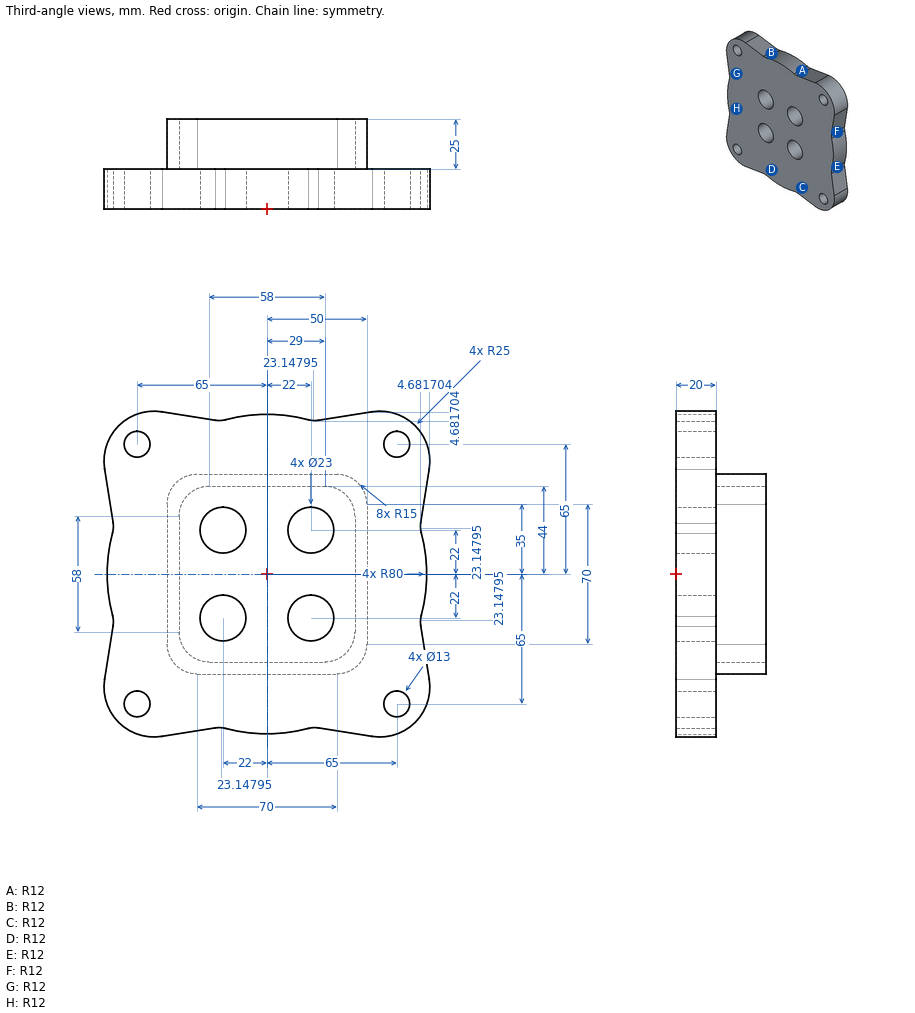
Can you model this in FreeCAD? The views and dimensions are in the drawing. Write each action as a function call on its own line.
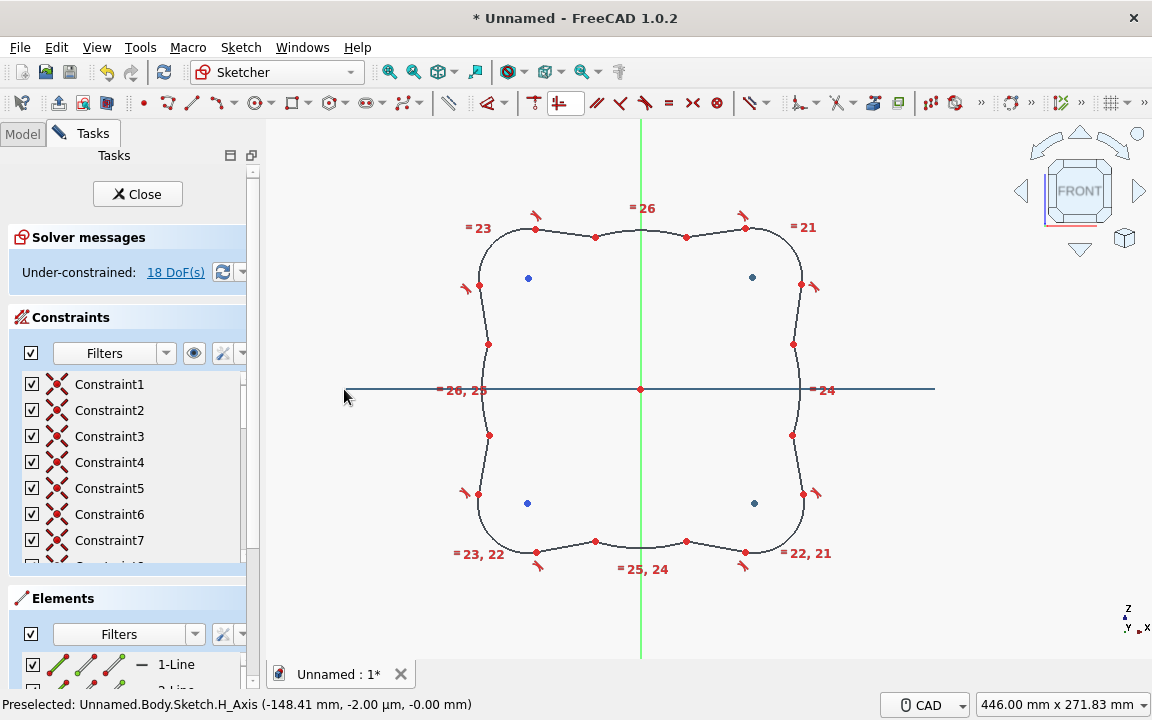
click(694, 104)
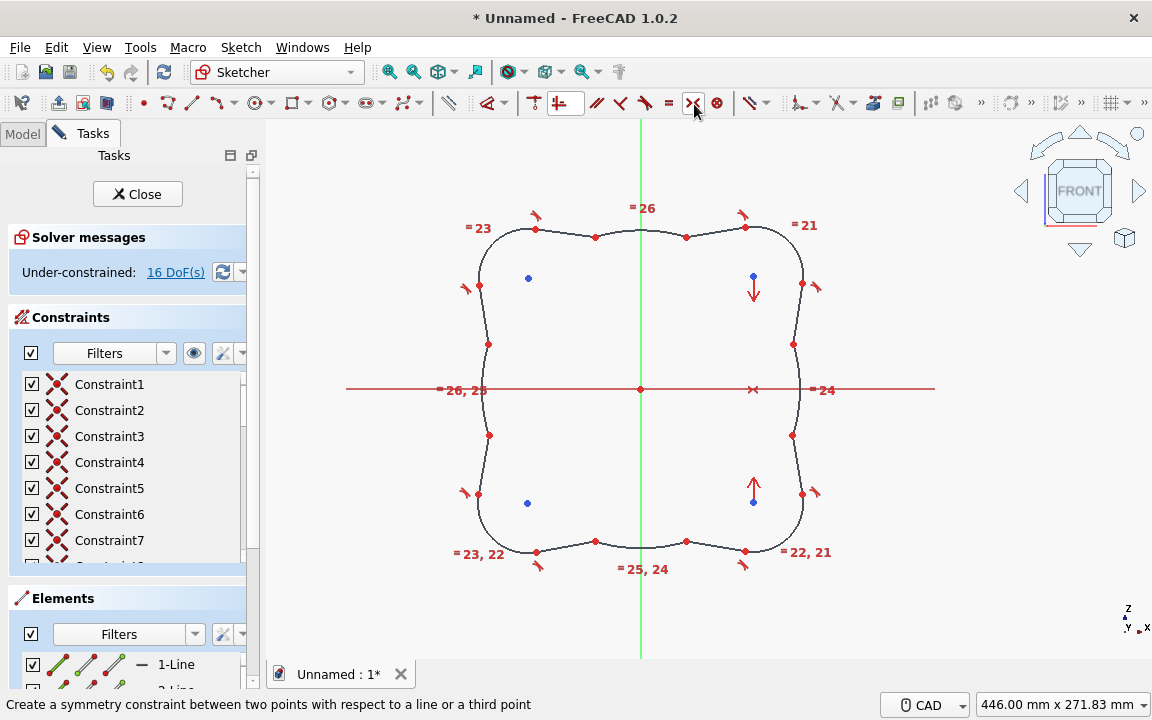
click(754, 502)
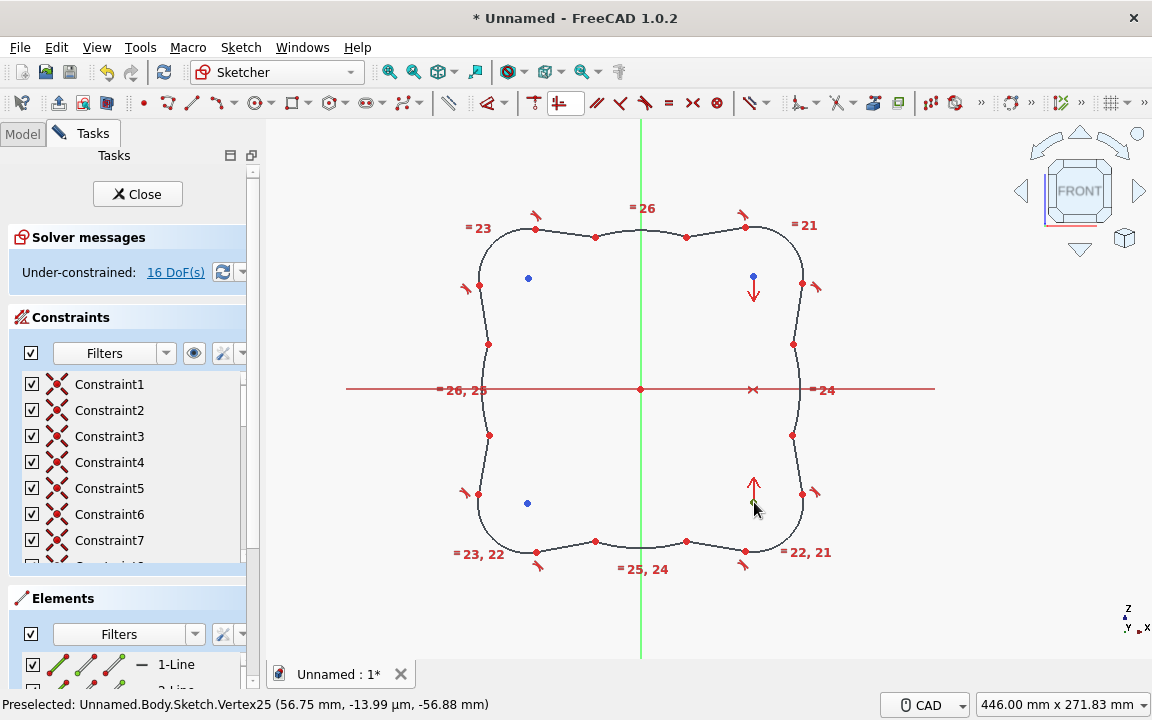
click(528, 504)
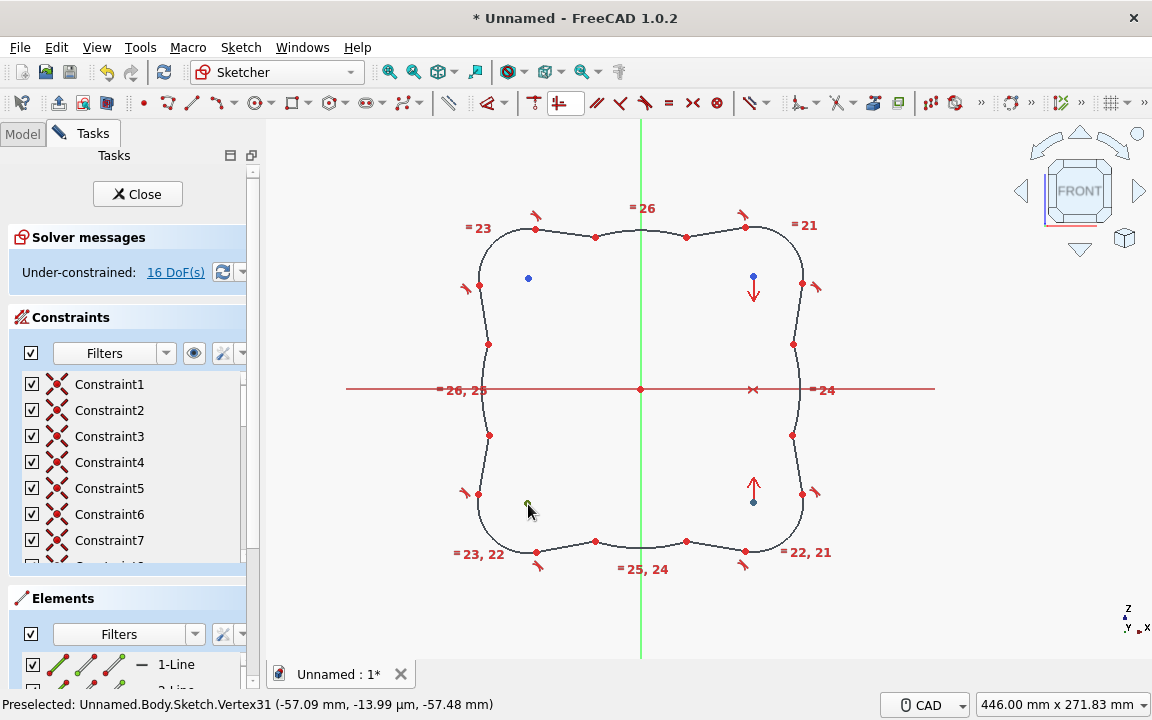
click(641, 596)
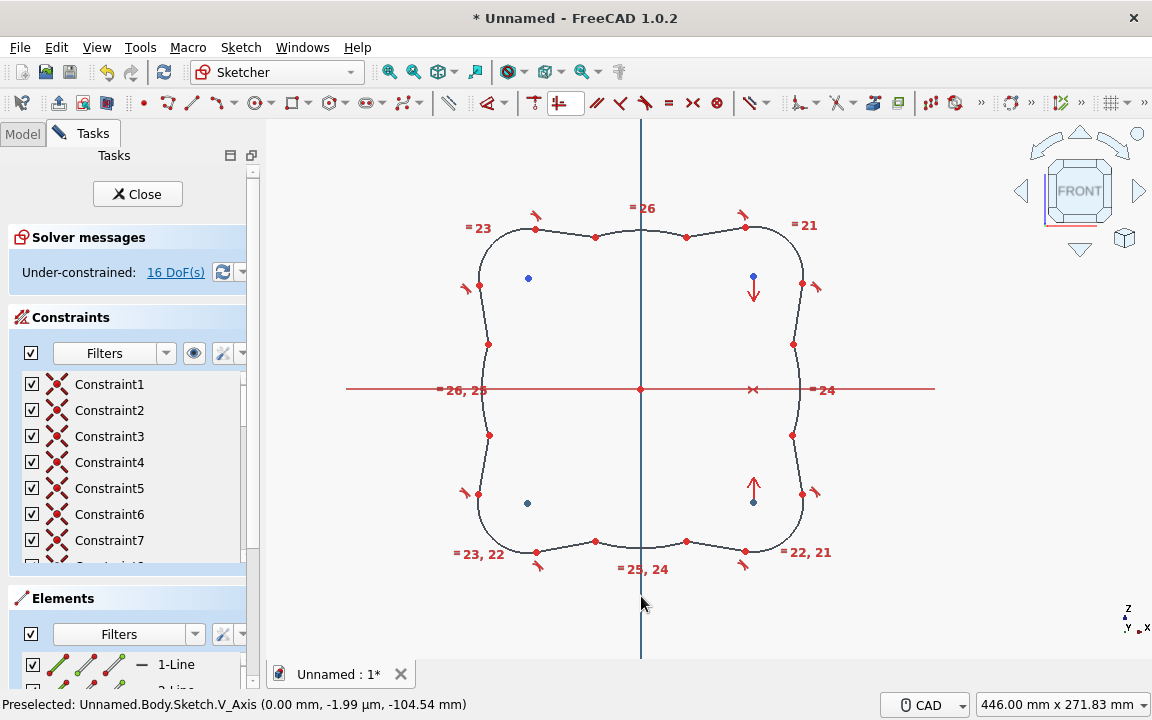
click(694, 104)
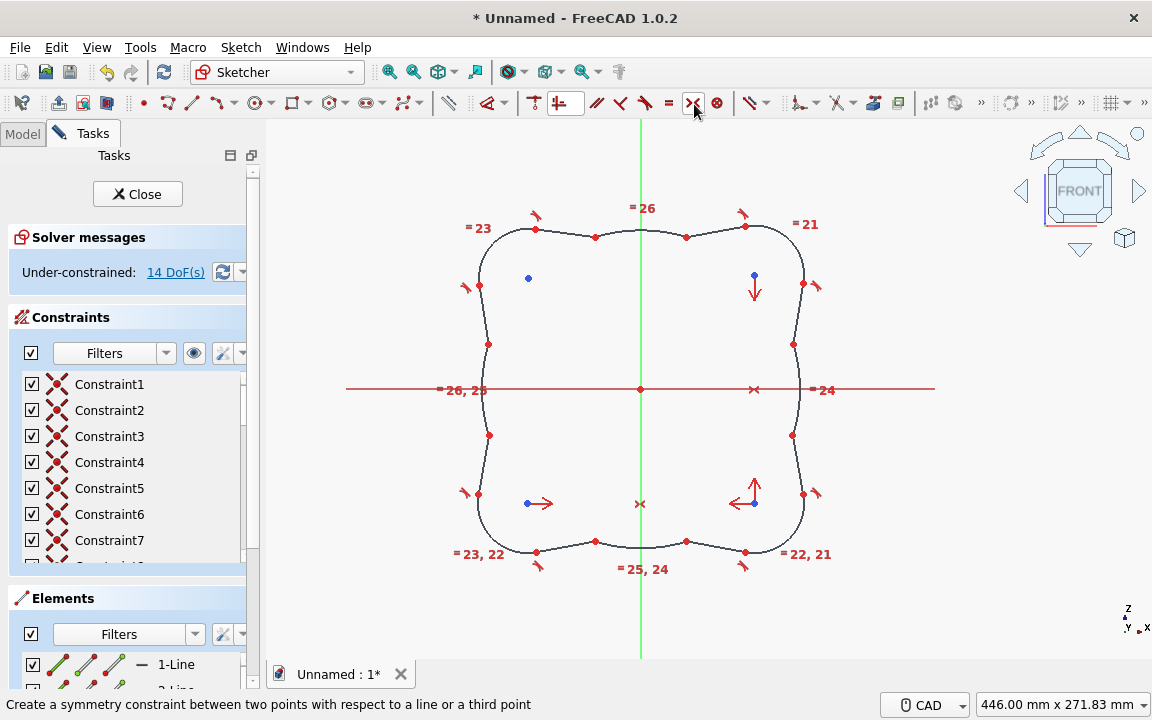
click(755, 275)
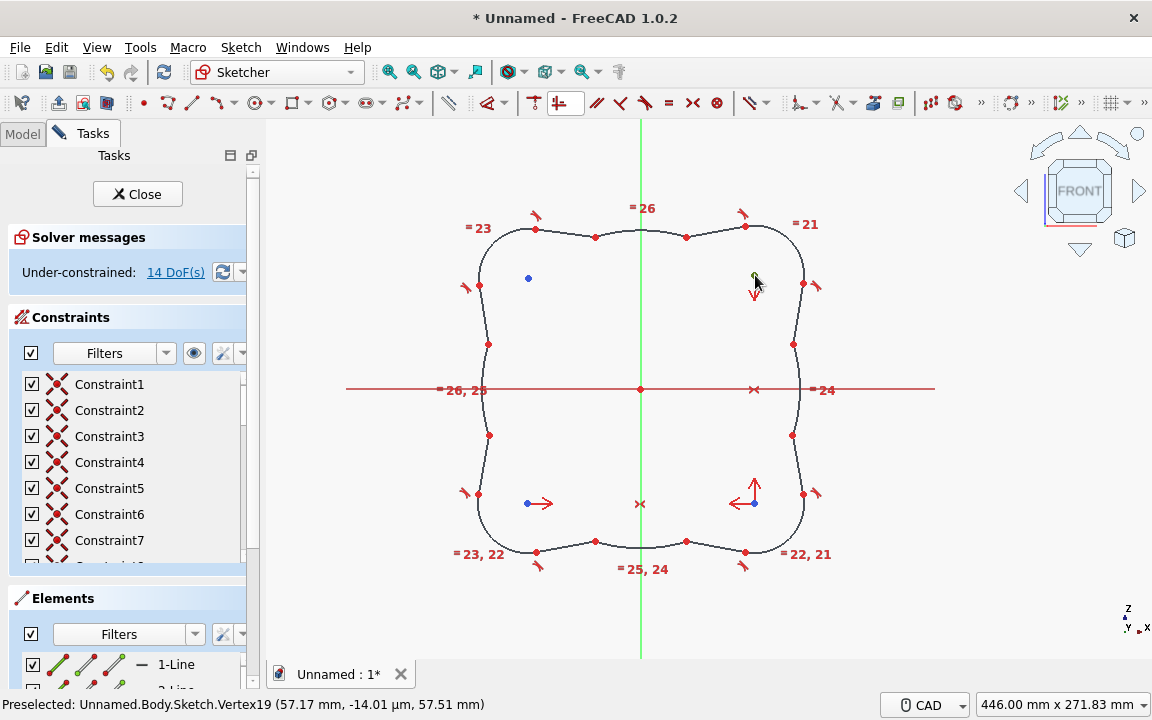
click(529, 278)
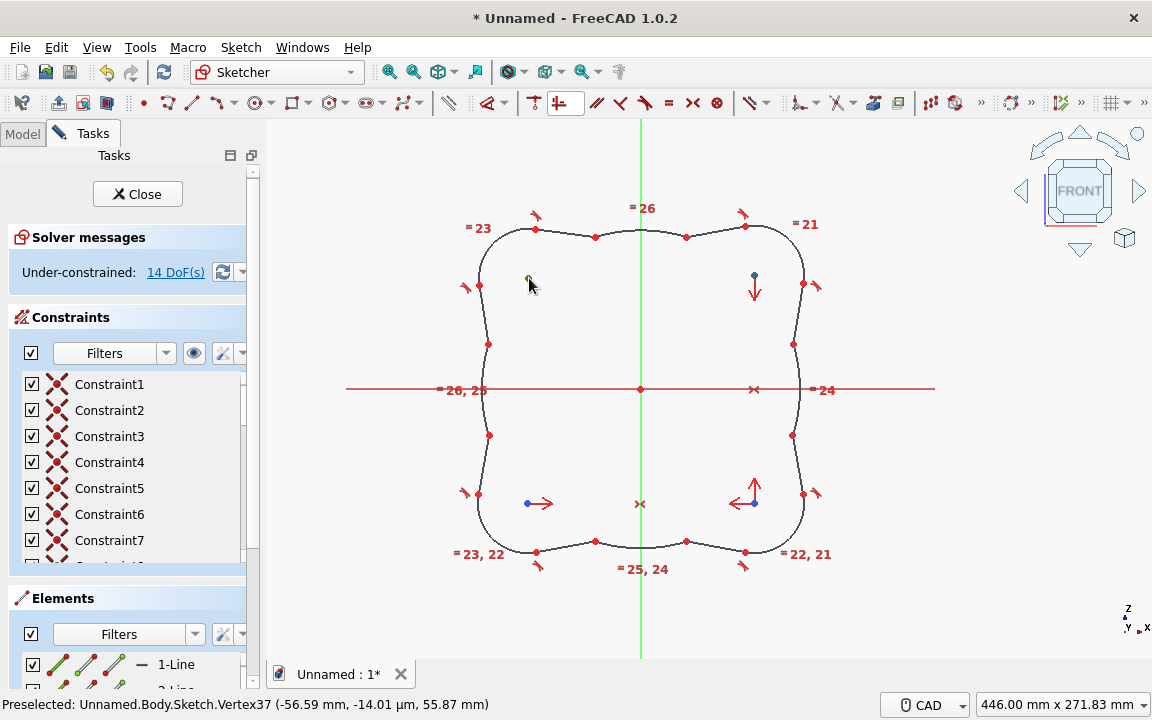
click(641, 596)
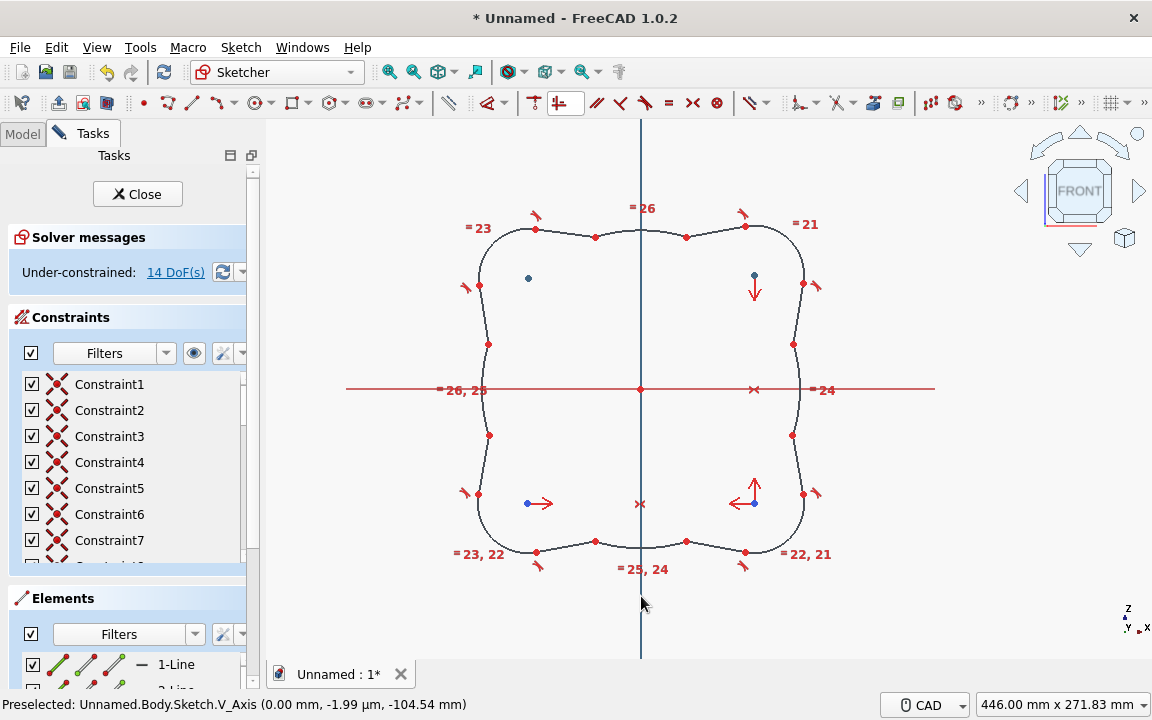
click(694, 104)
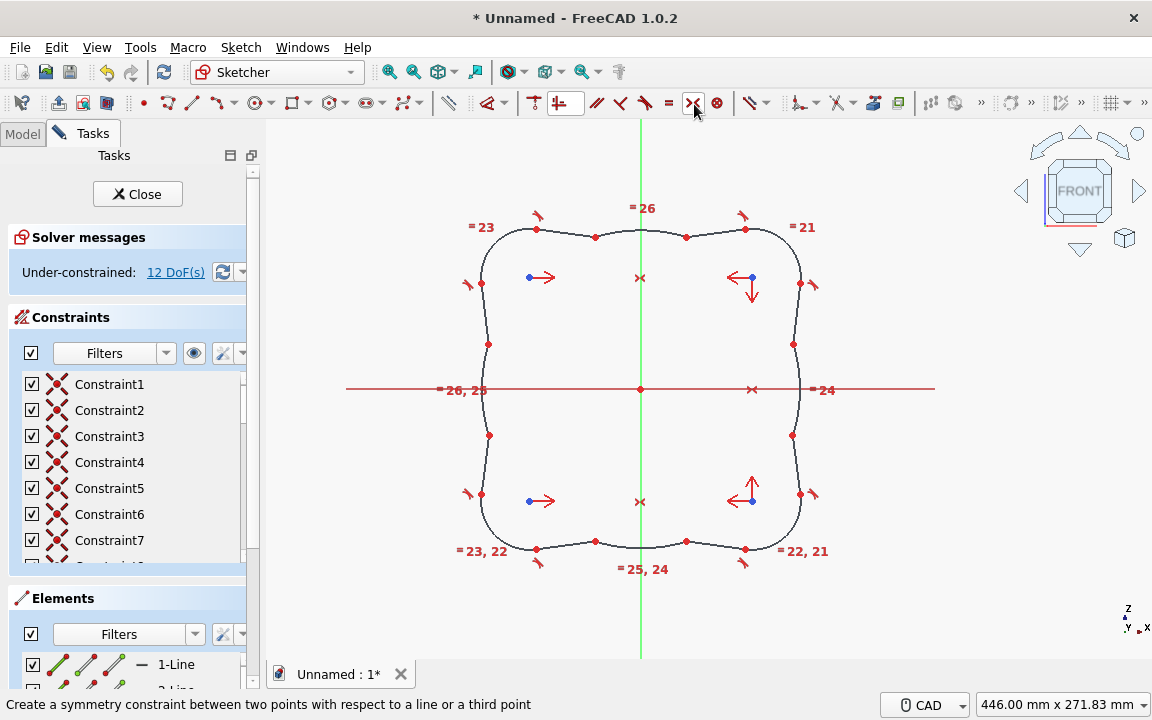
click(488, 104)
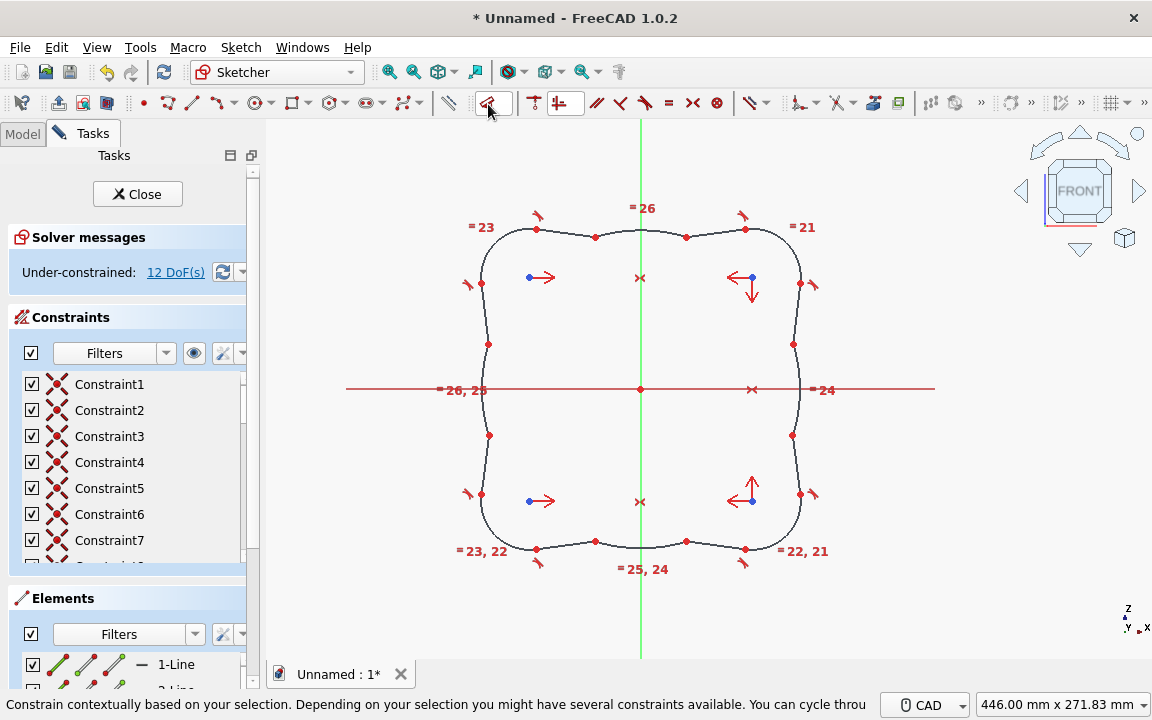
click(796, 257)
click(825, 243)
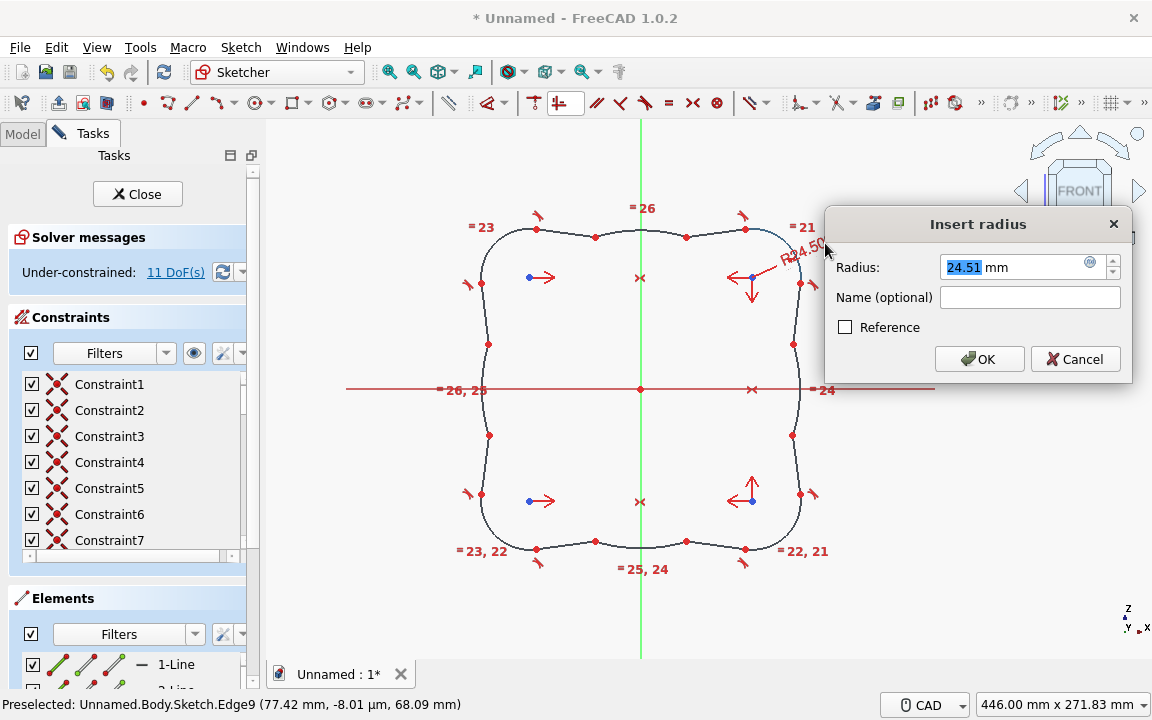
text(25)
key(Return)